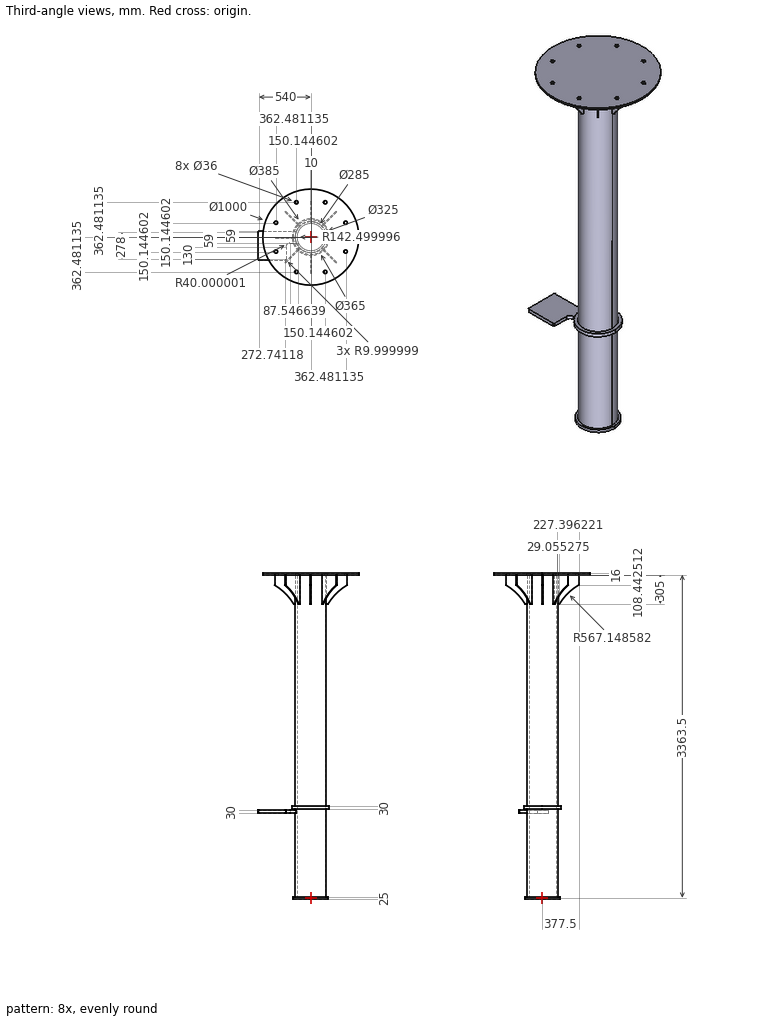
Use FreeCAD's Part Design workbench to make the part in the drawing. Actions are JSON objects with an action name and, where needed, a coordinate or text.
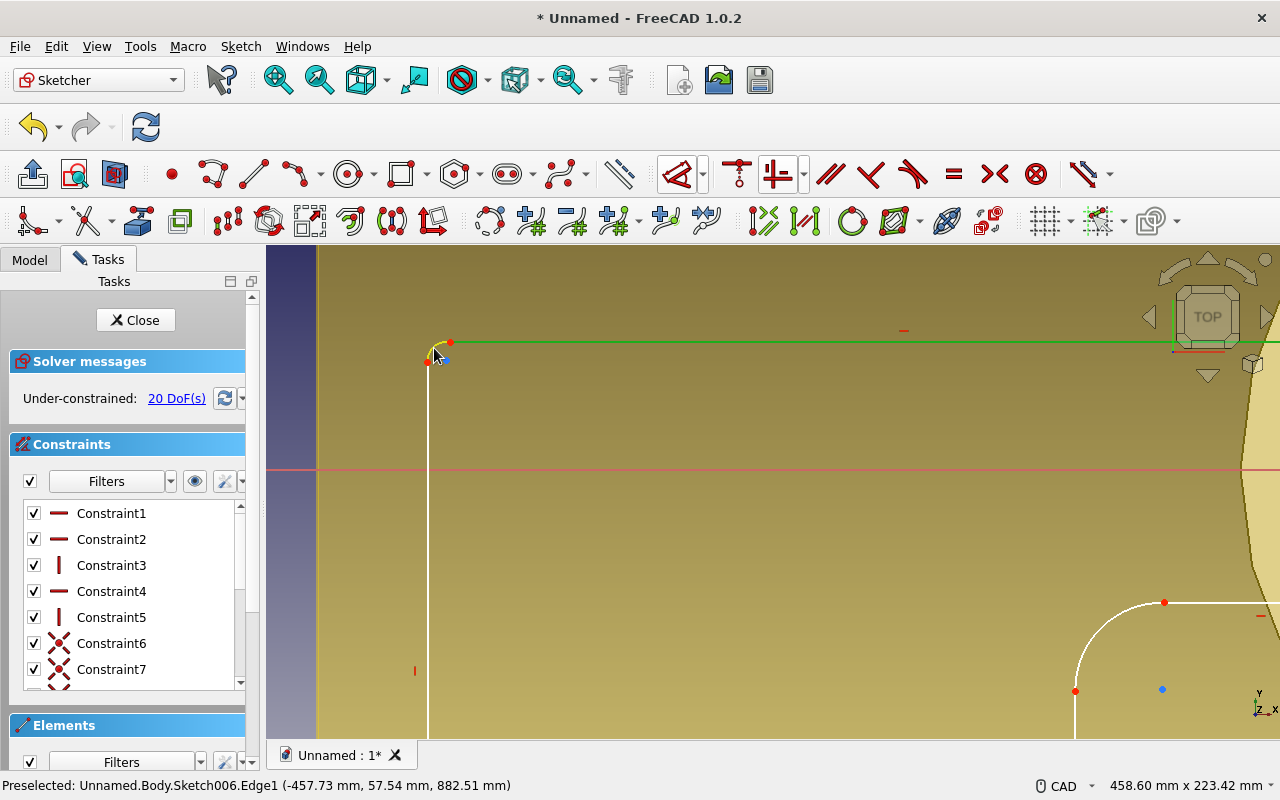
{"action": "left_click", "coordinate": [434, 347]}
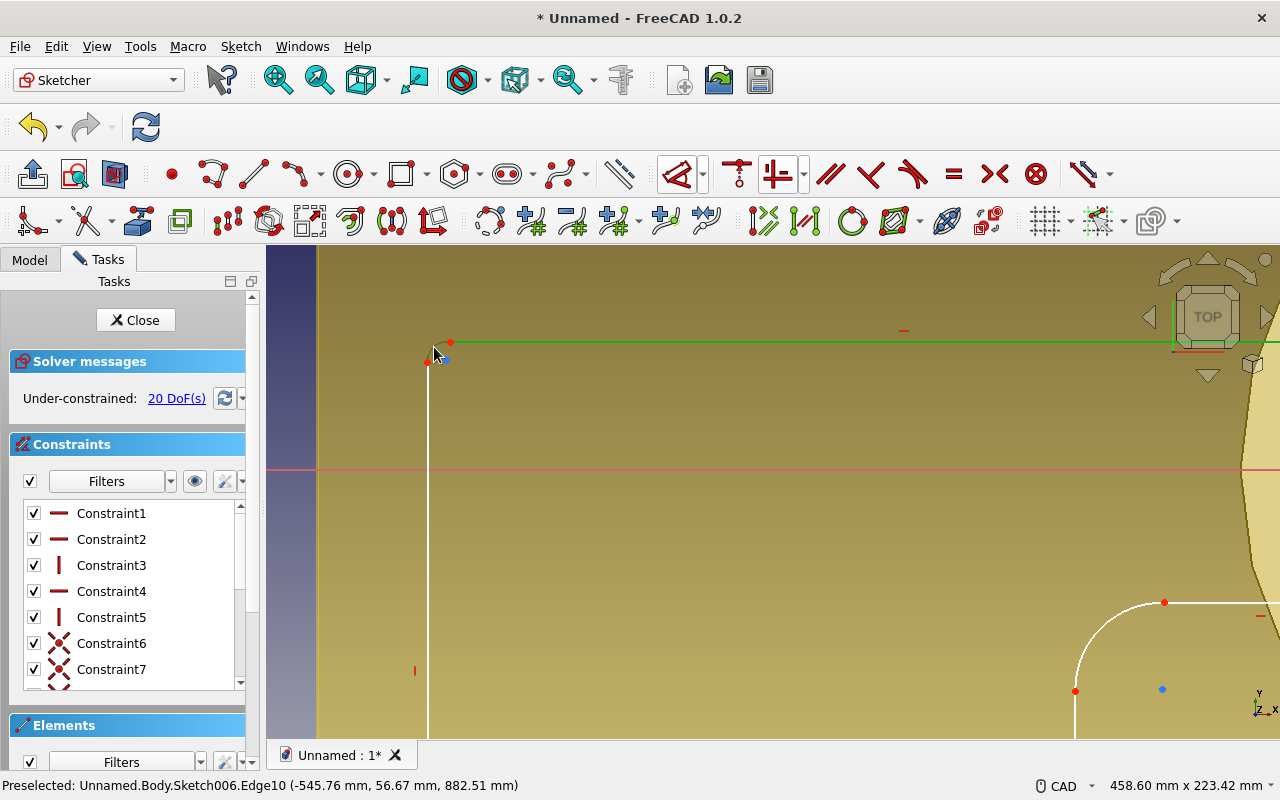
{"action": "key", "text": "t"}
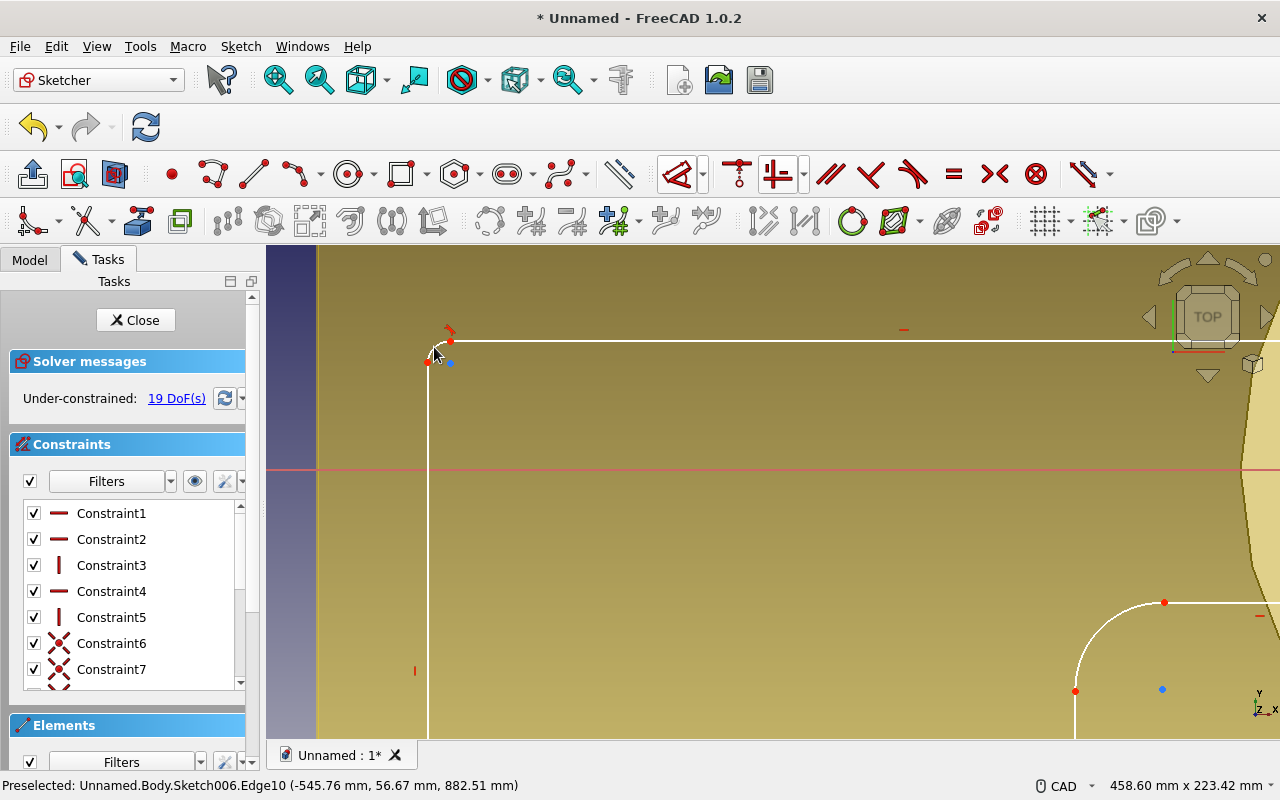
{"action": "scroll", "coordinate": [434, 348], "scroll_direction": "down", "scroll_amount": 4}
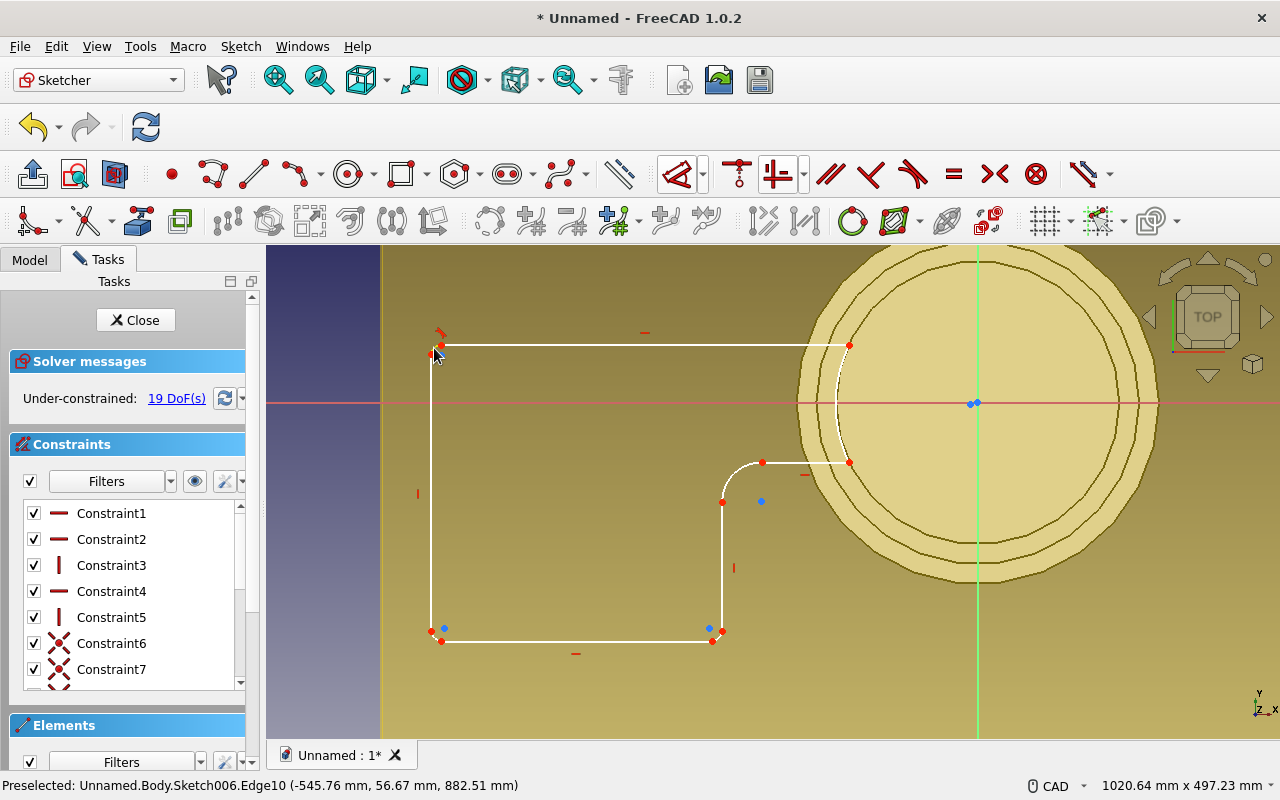
{"action": "left_click", "coordinate": [722, 541]}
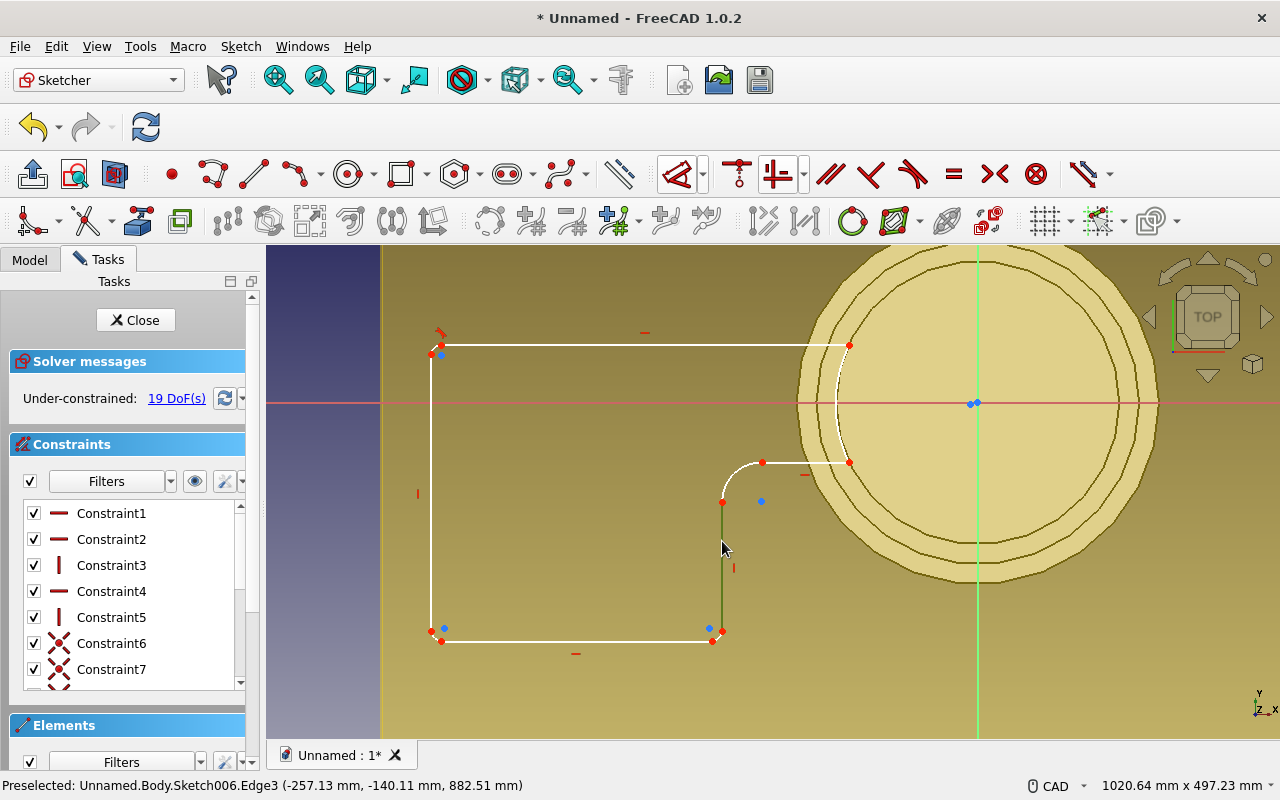
{"action": "scroll", "coordinate": [719, 638], "scroll_direction": "up", "scroll_amount": 4}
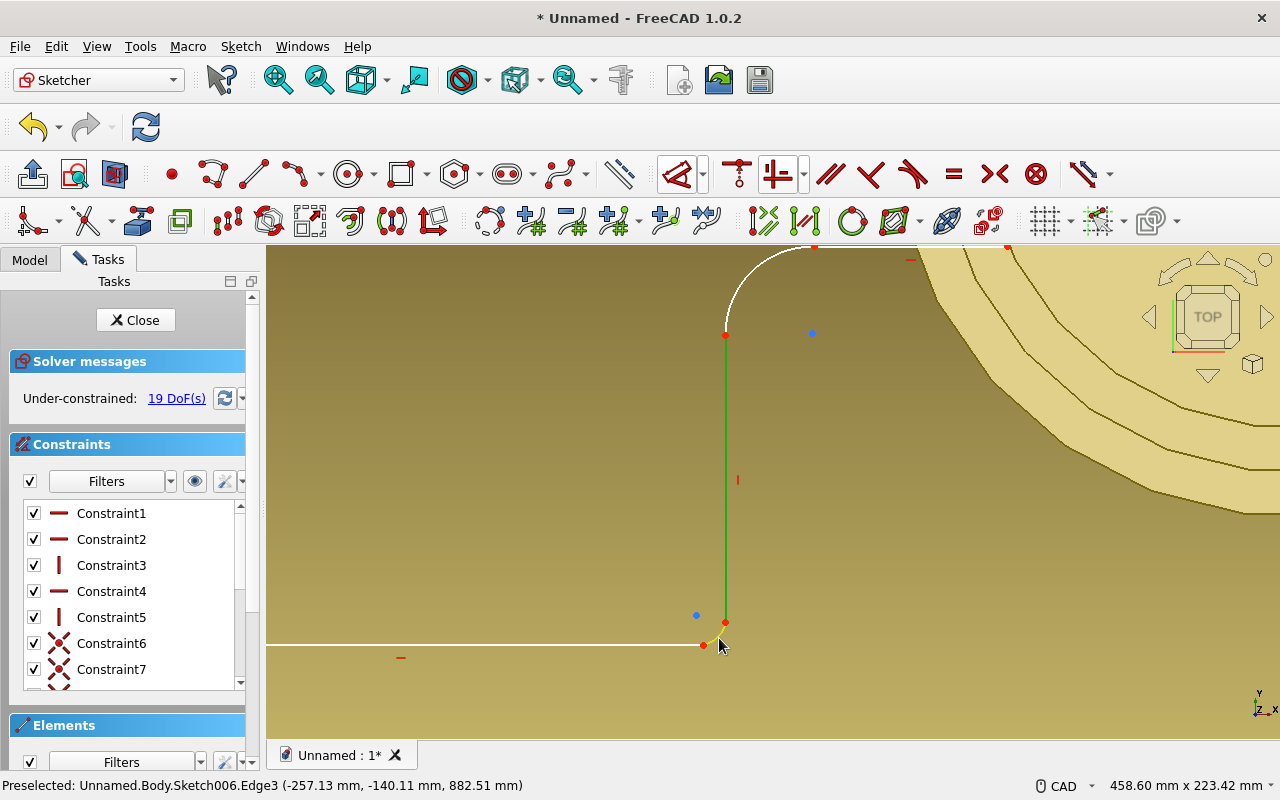
{"action": "left_click", "coordinate": [718, 637]}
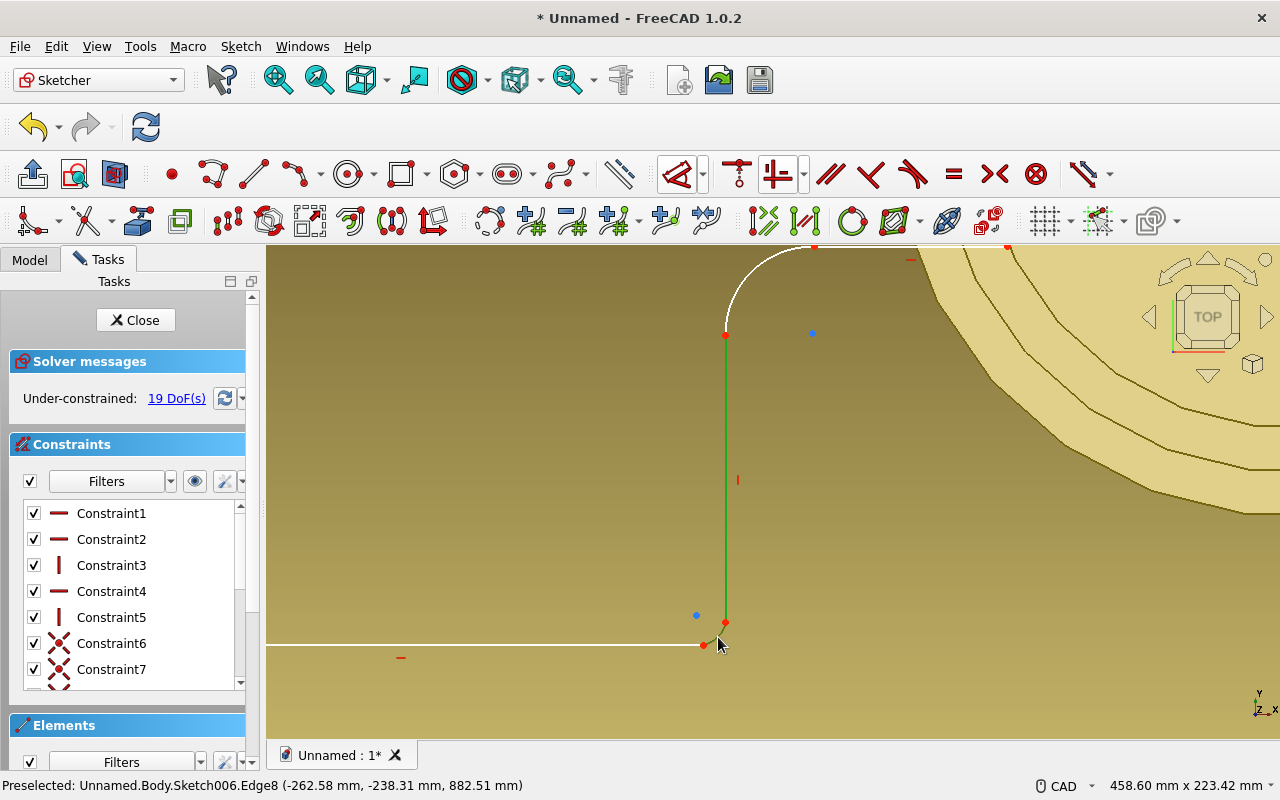
{"action": "key", "text": "t"}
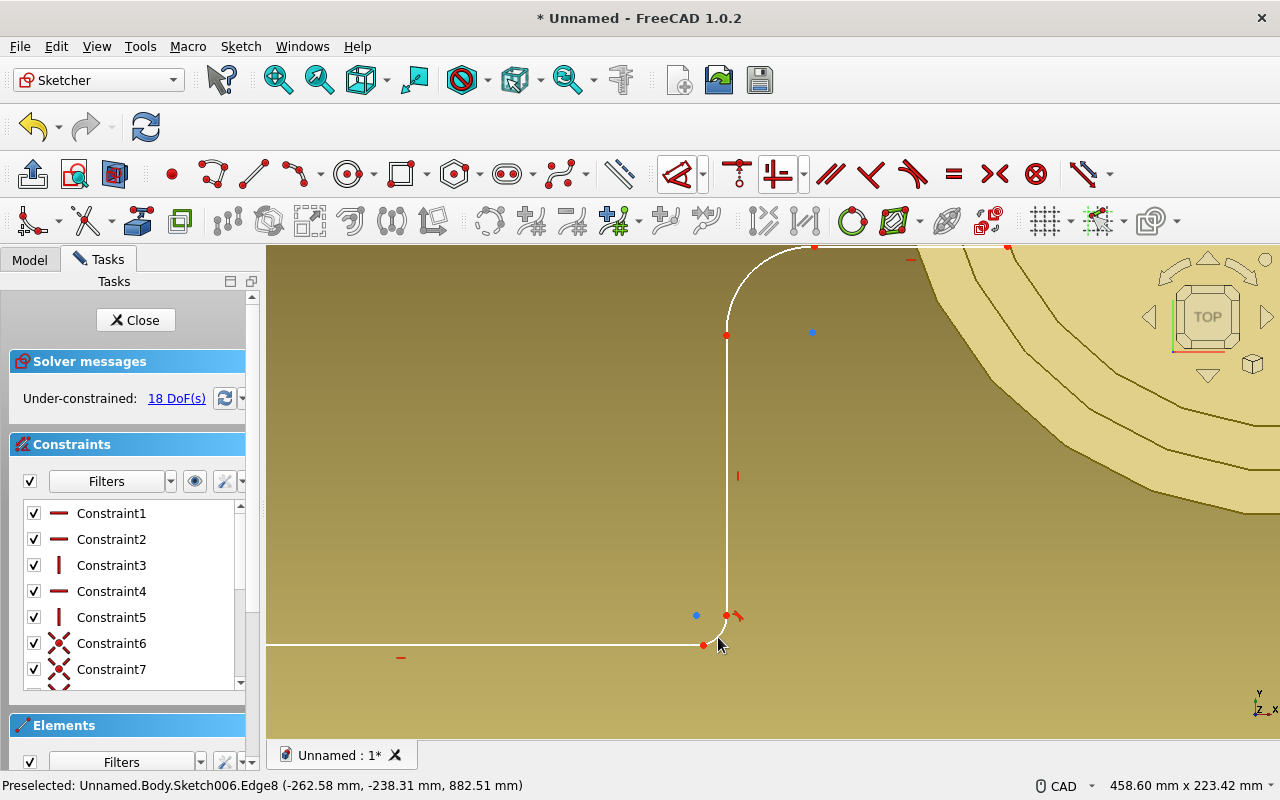
{"action": "left_click", "coordinate": [523, 645]}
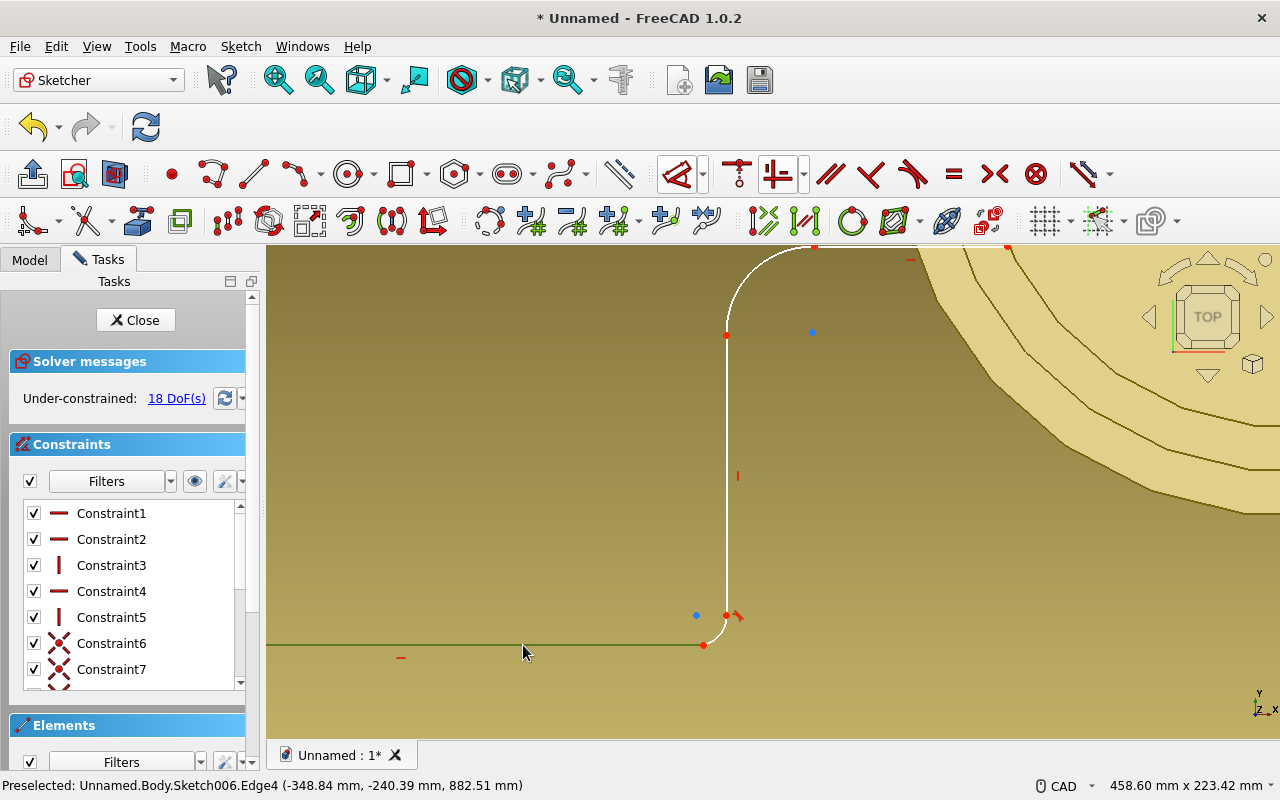
{"action": "left_click", "coordinate": [714, 640]}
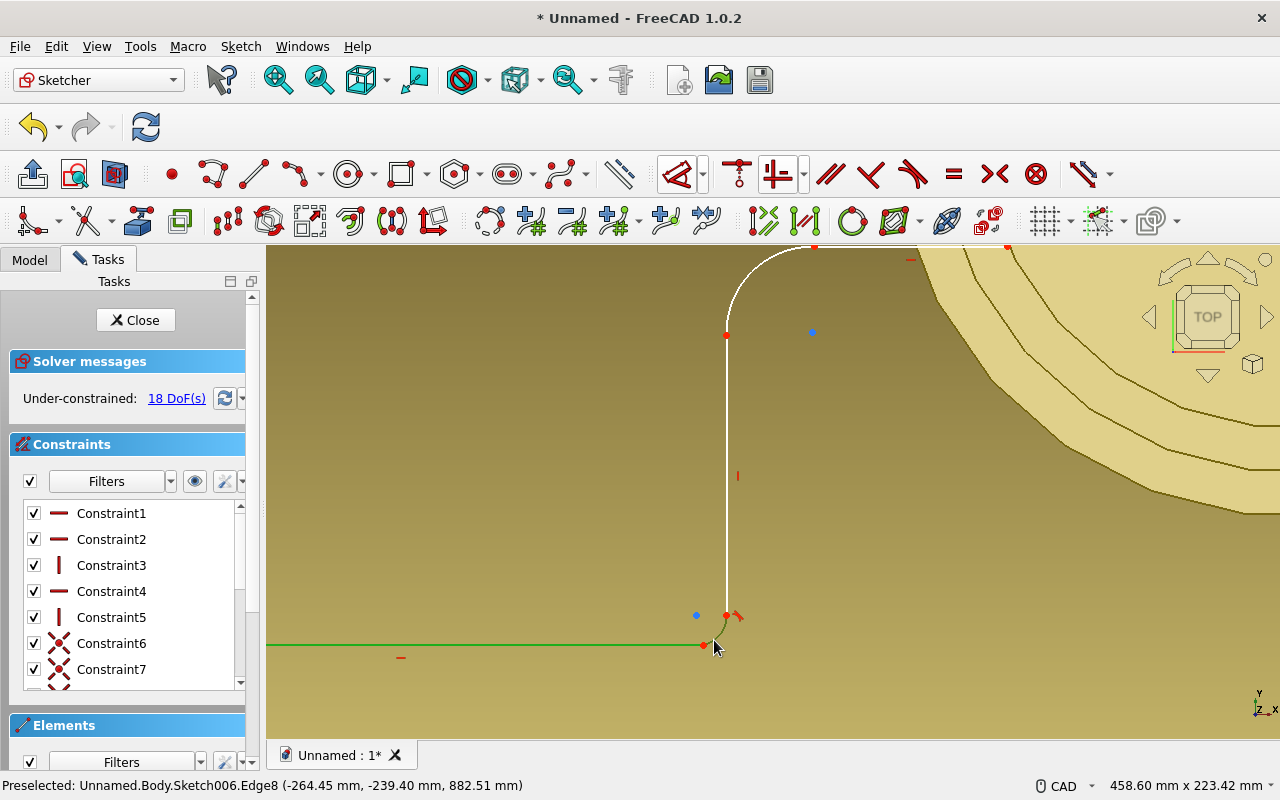
{"action": "left_click", "coordinate": [913, 174]}